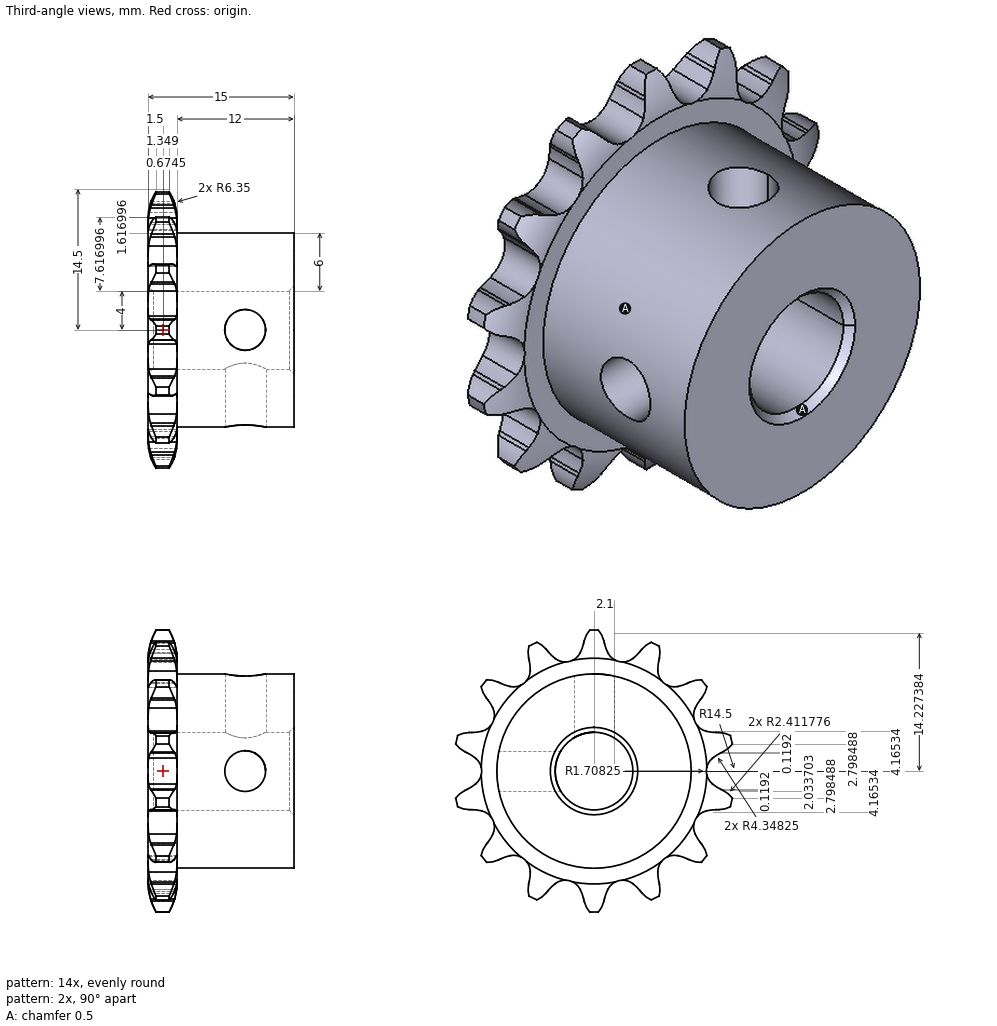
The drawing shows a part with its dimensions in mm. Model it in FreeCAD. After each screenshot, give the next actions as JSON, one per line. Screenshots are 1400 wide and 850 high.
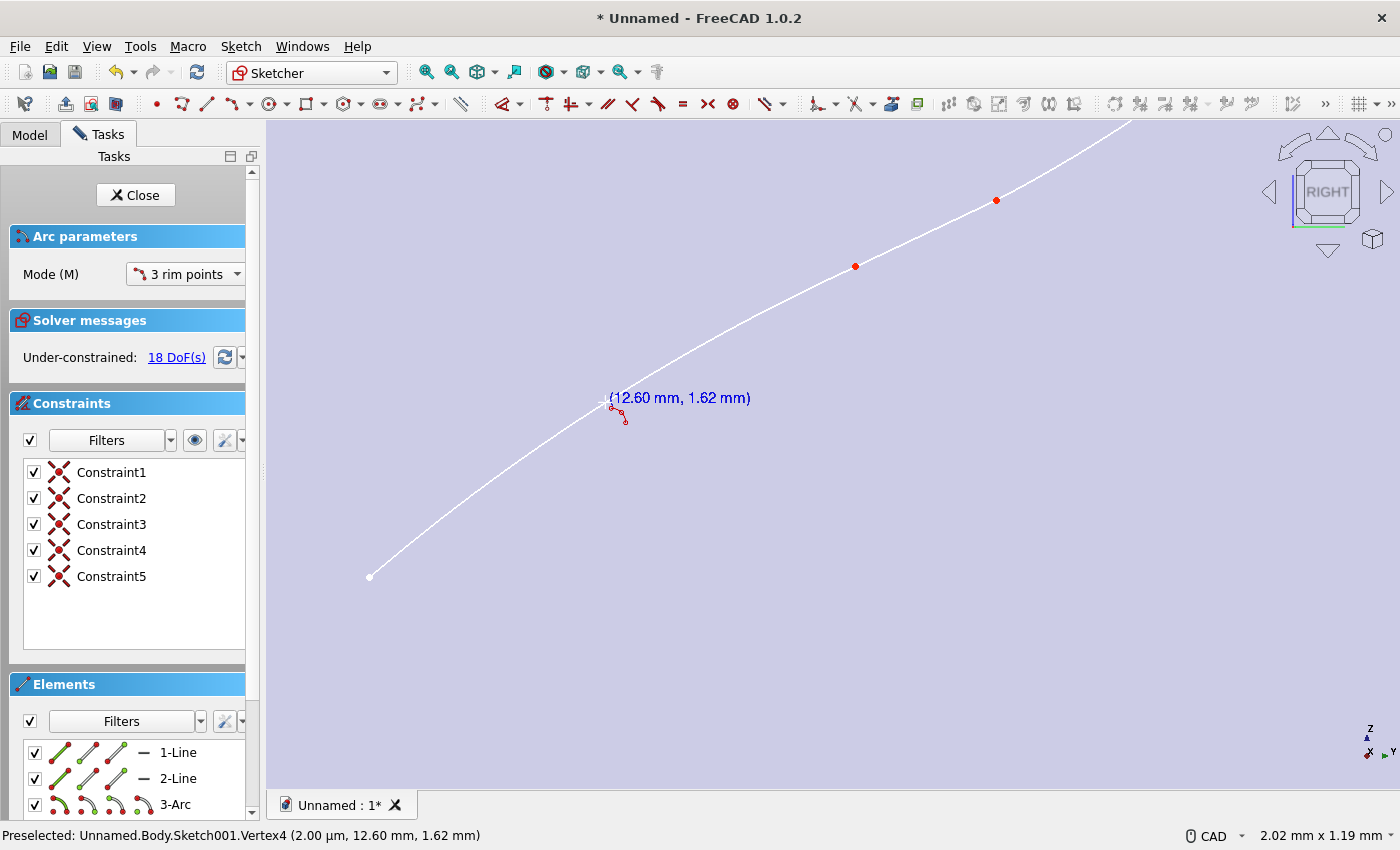
{"action": "scroll", "coordinate": [752, 320], "scroll_direction": "down", "scroll_amount": 10}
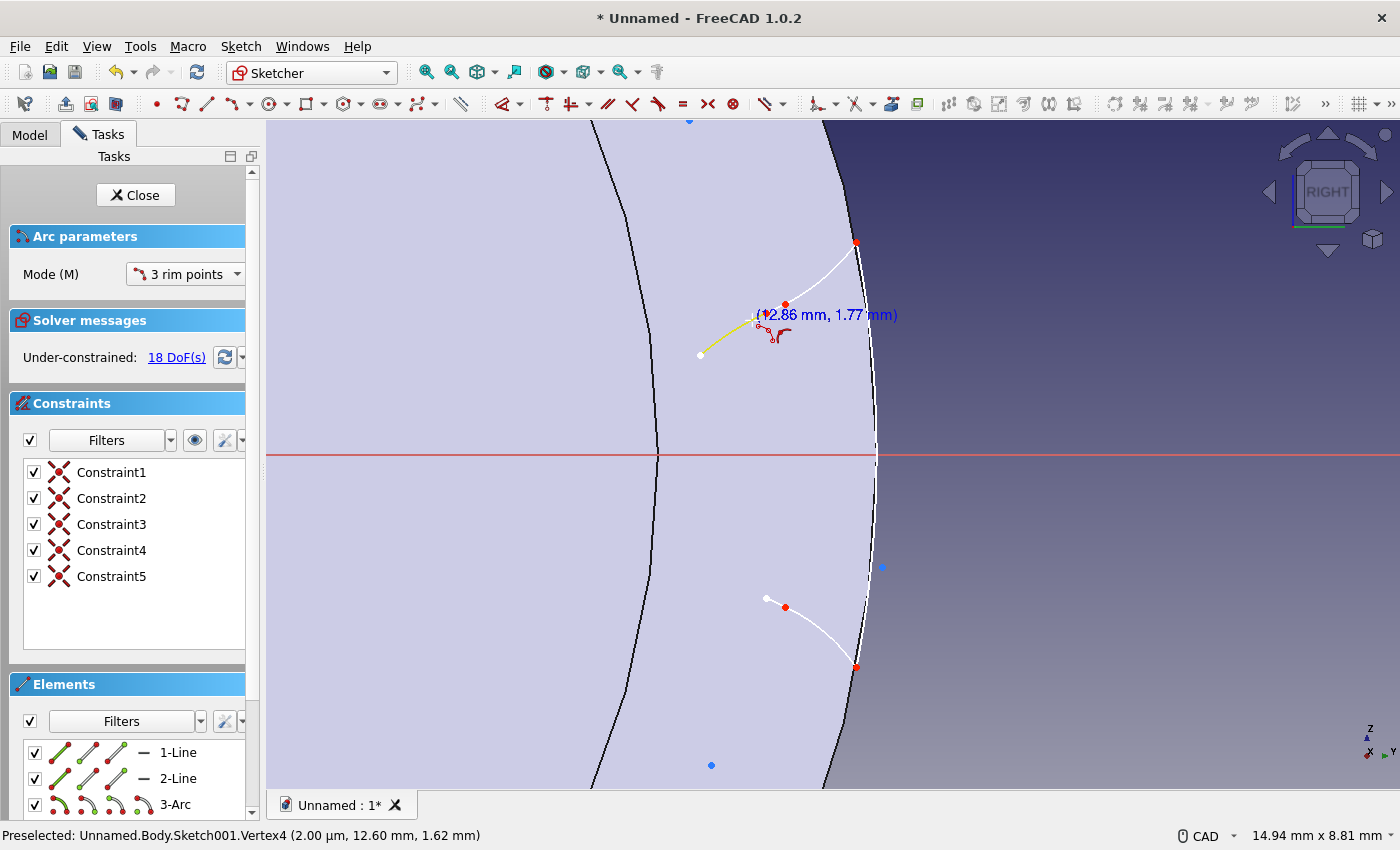
{"action": "left_click", "coordinate": [701, 355]}
{"action": "left_click", "coordinate": [701, 554]}
{"action": "left_click", "coordinate": [656, 432]}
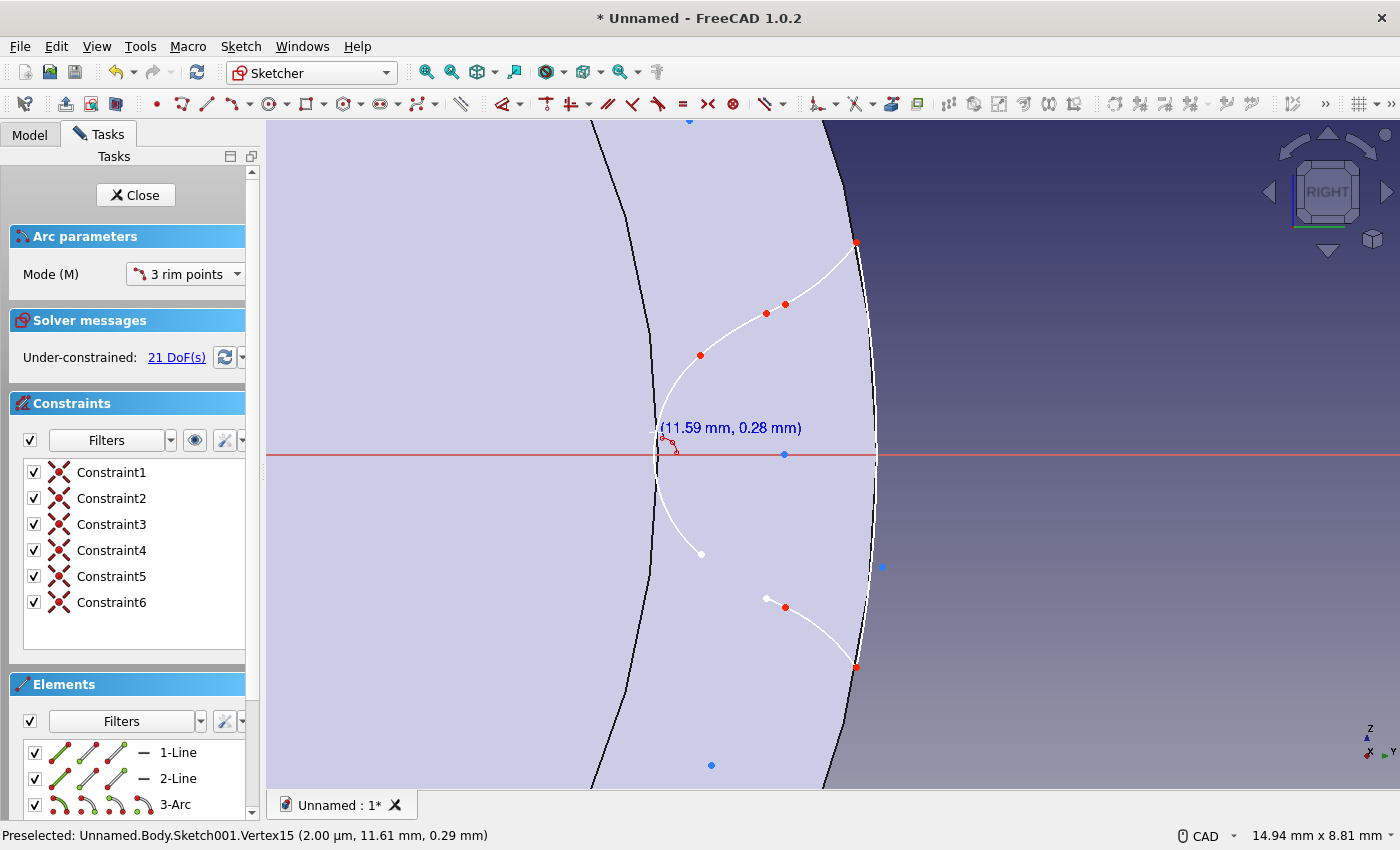
{"action": "left_click", "coordinate": [701, 555]}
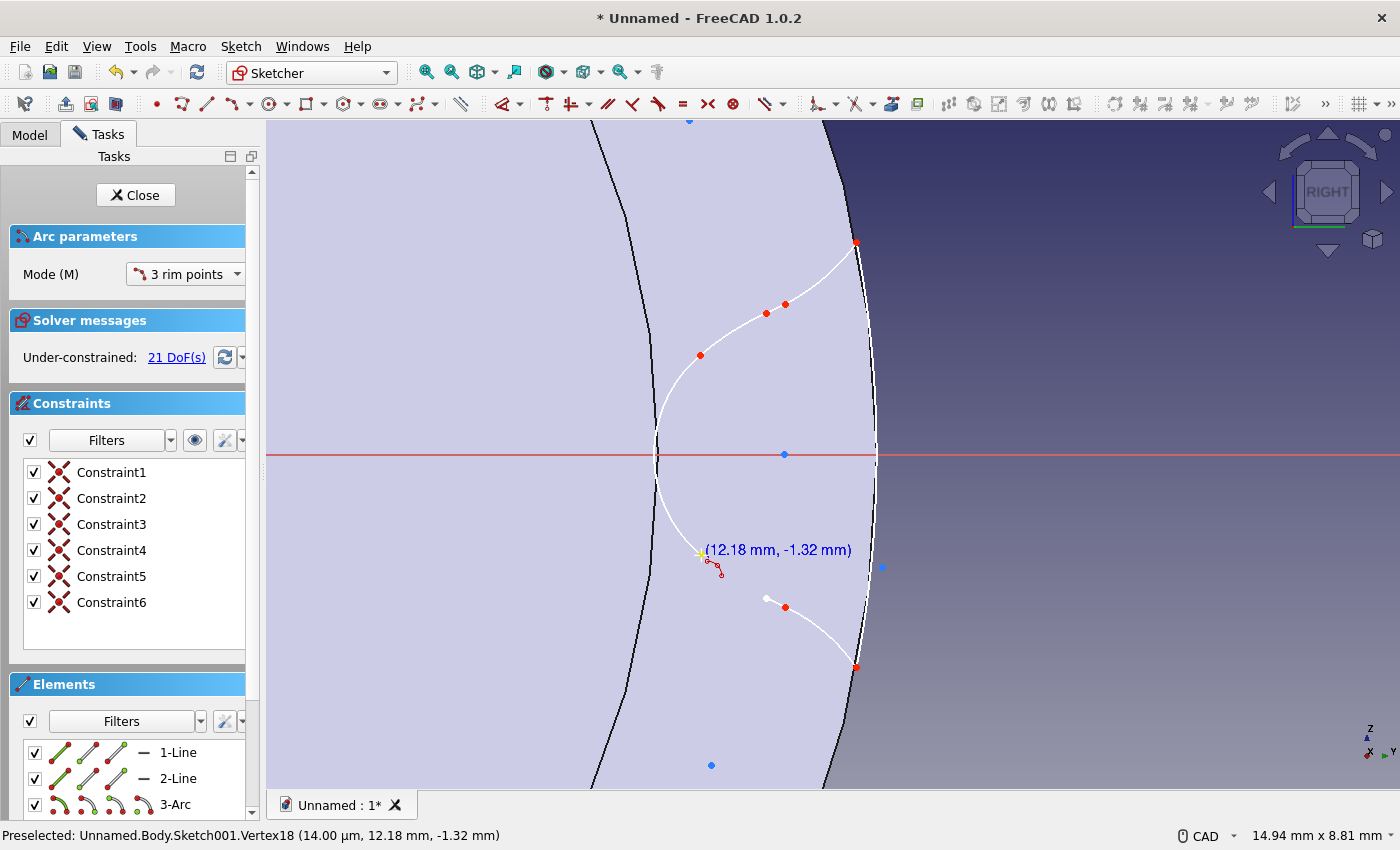
{"action": "scroll", "coordinate": [767, 597], "scroll_direction": "up", "scroll_amount": 3}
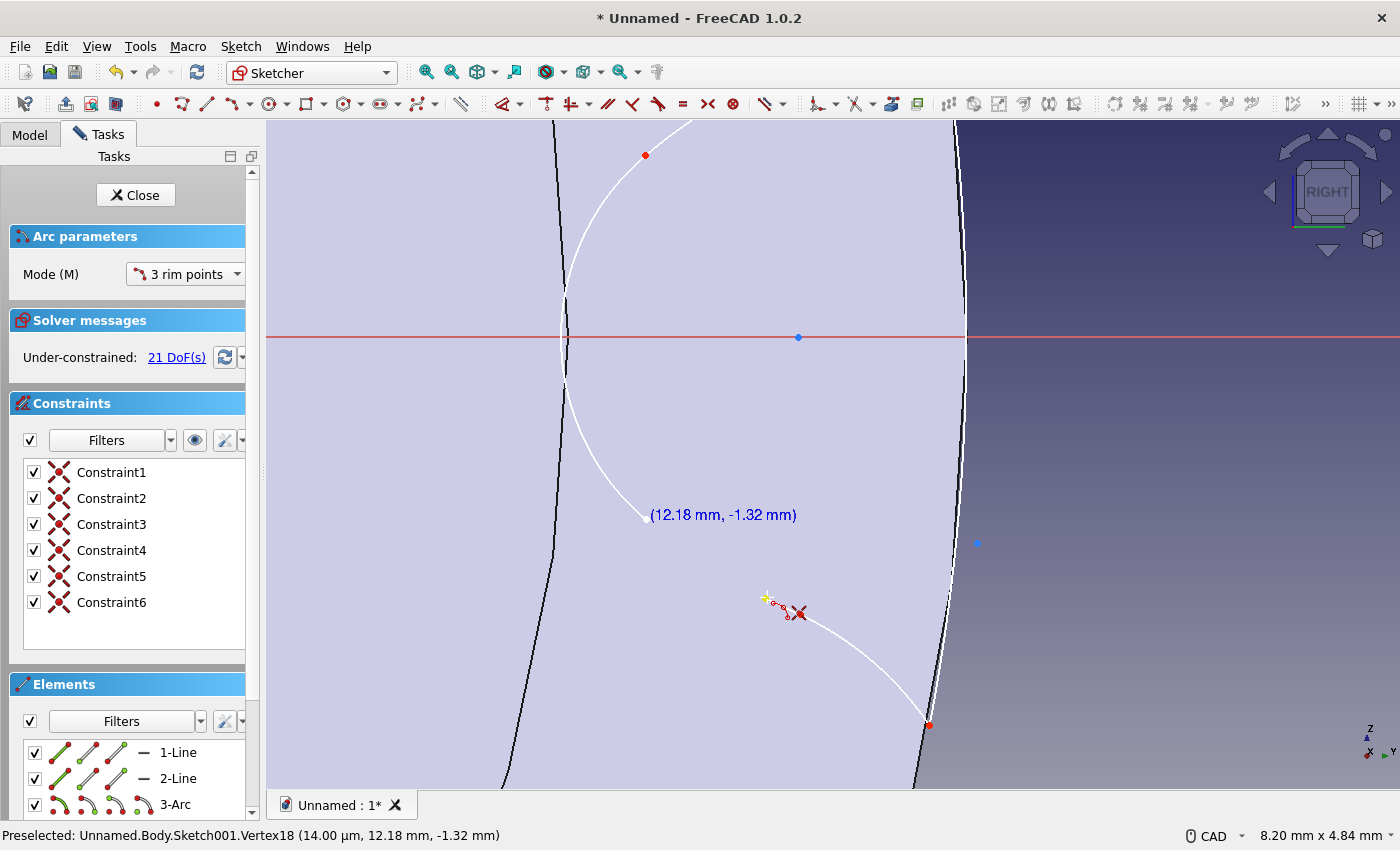
{"action": "left_click", "coordinate": [766, 598]}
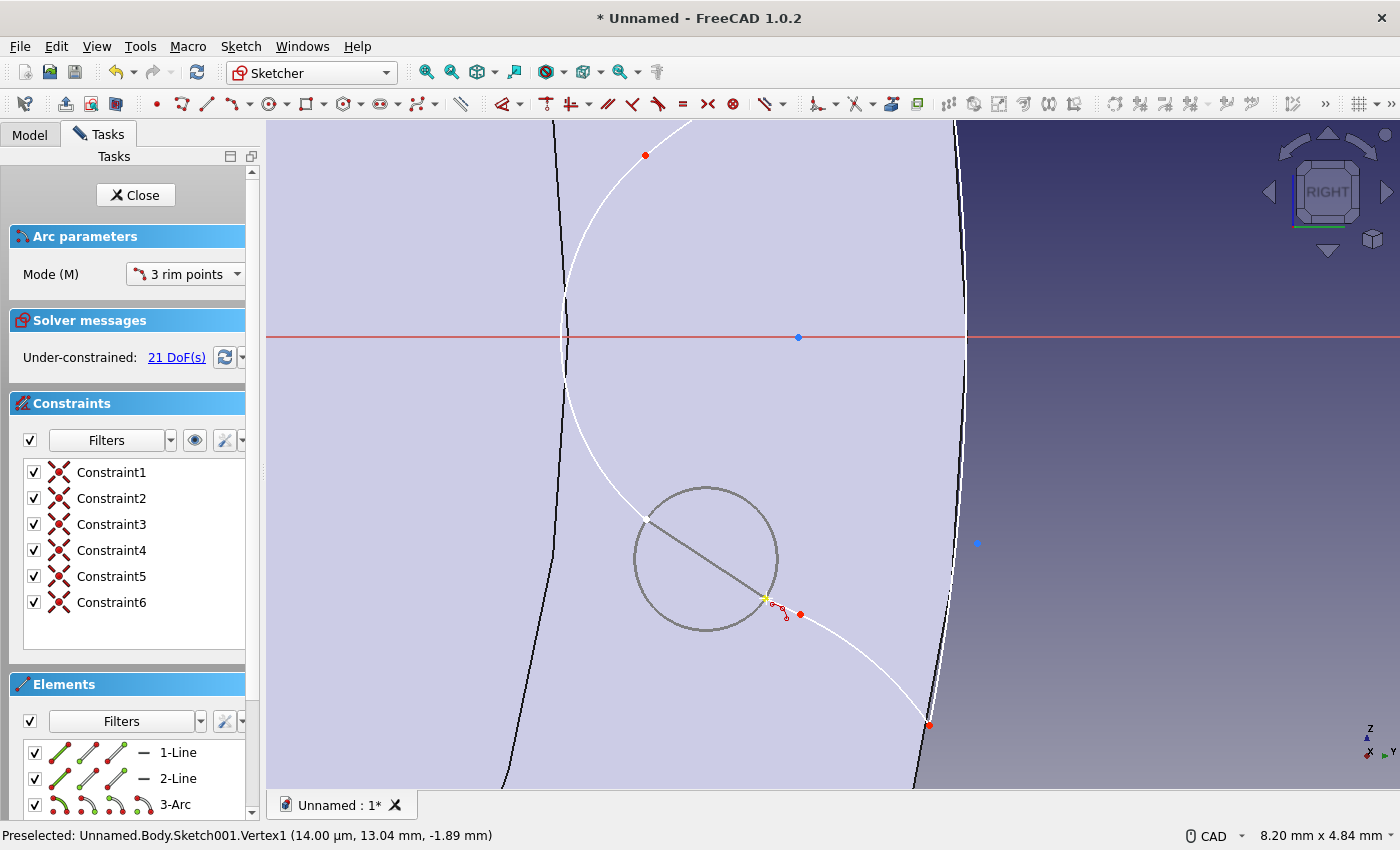
{"action": "scroll", "coordinate": [704, 561], "scroll_direction": "up", "scroll_amount": 7}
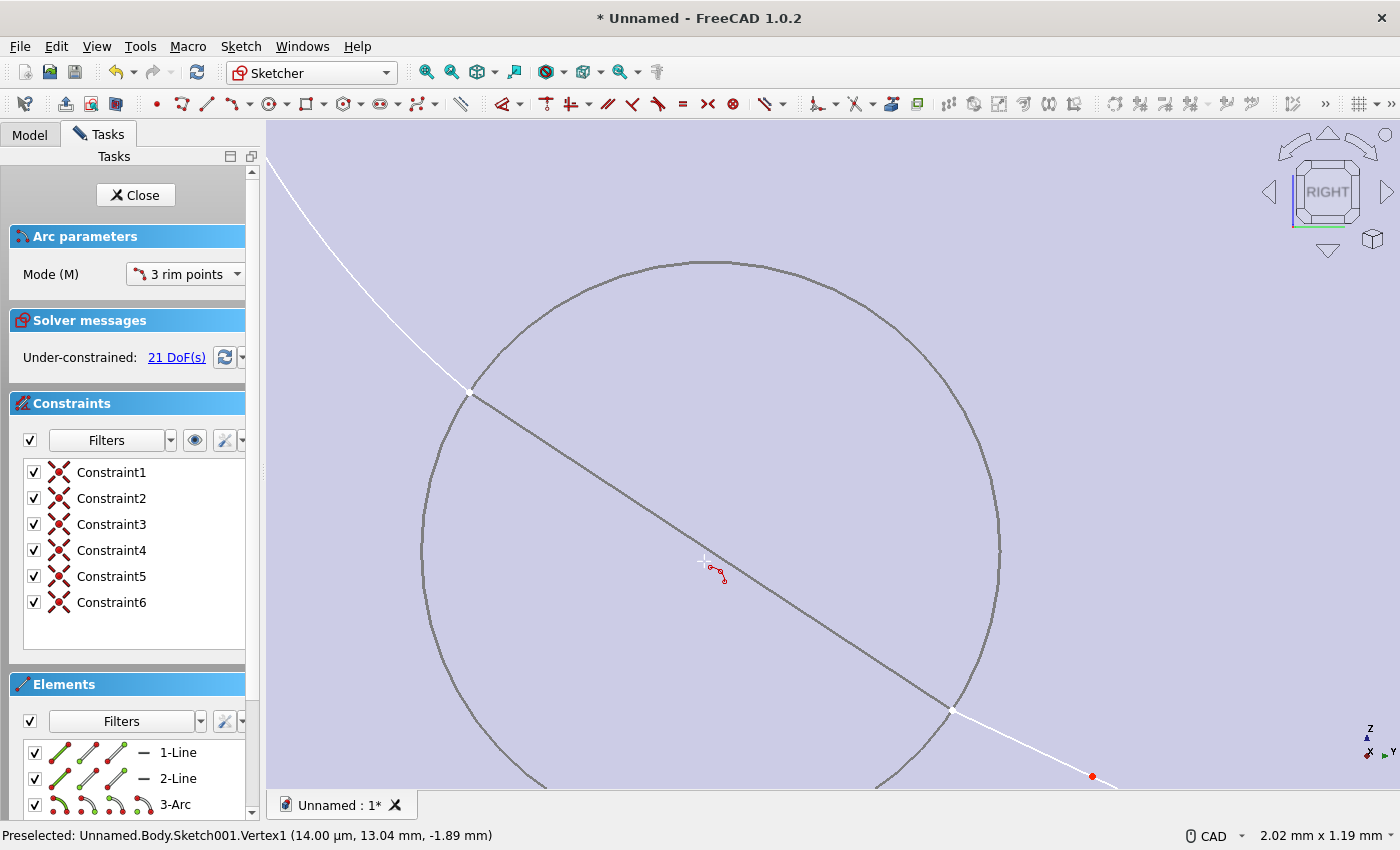
{"action": "left_click", "coordinate": [701, 560]}
{"action": "key", "text": "Escape"}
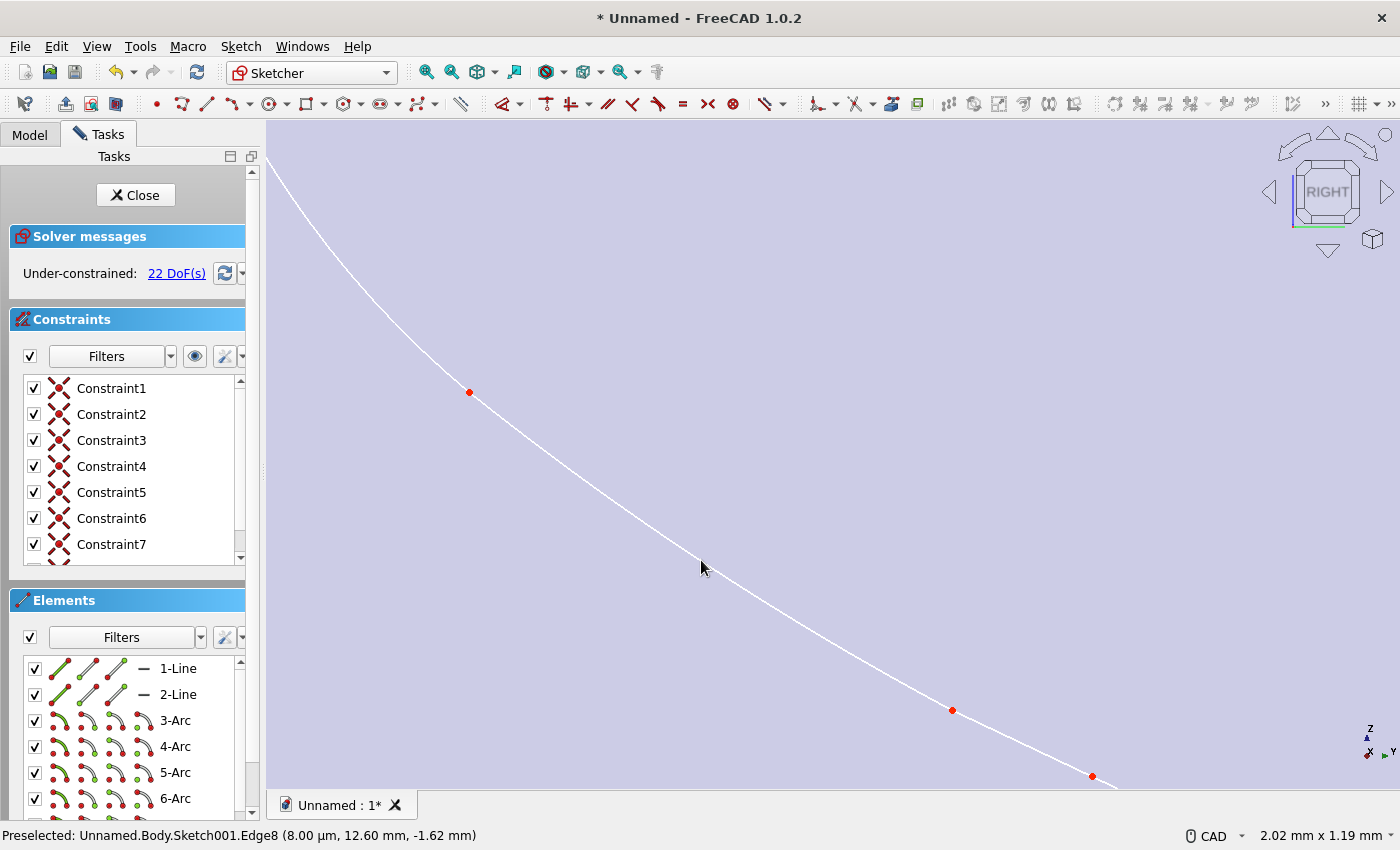
{"action": "scroll", "coordinate": [736, 580], "scroll_direction": "down", "scroll_amount": 10}